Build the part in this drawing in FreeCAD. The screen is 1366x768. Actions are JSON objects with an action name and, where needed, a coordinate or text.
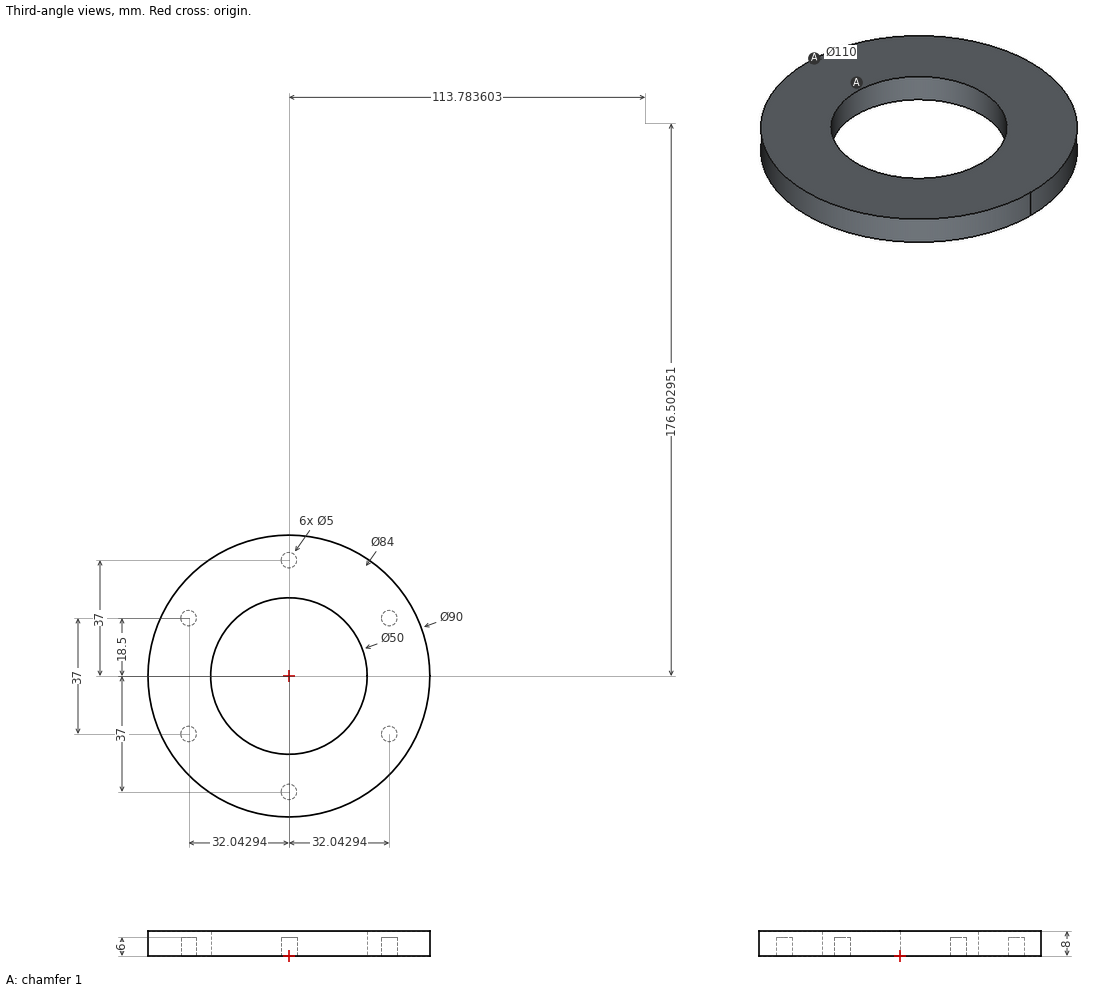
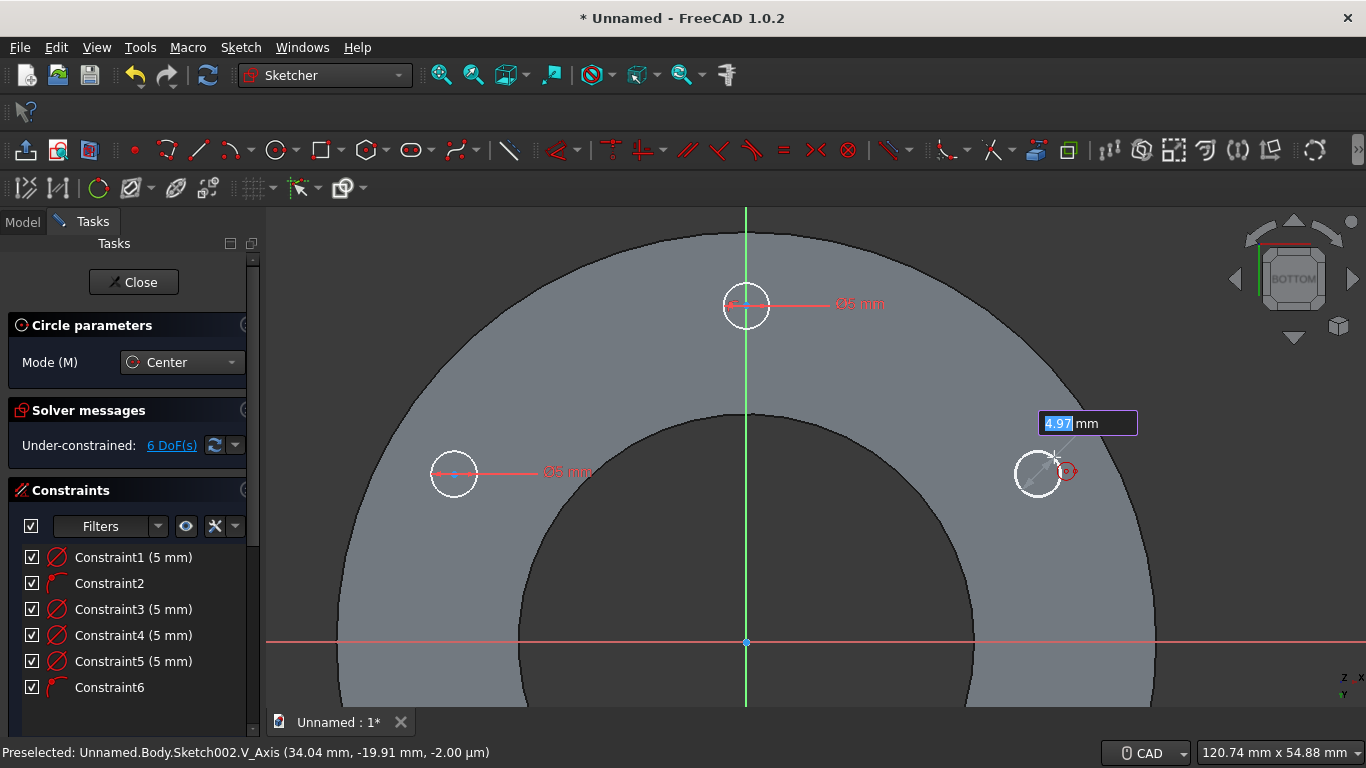
{"action": "type", "text": "5"}
{"action": "key", "text": "Return"}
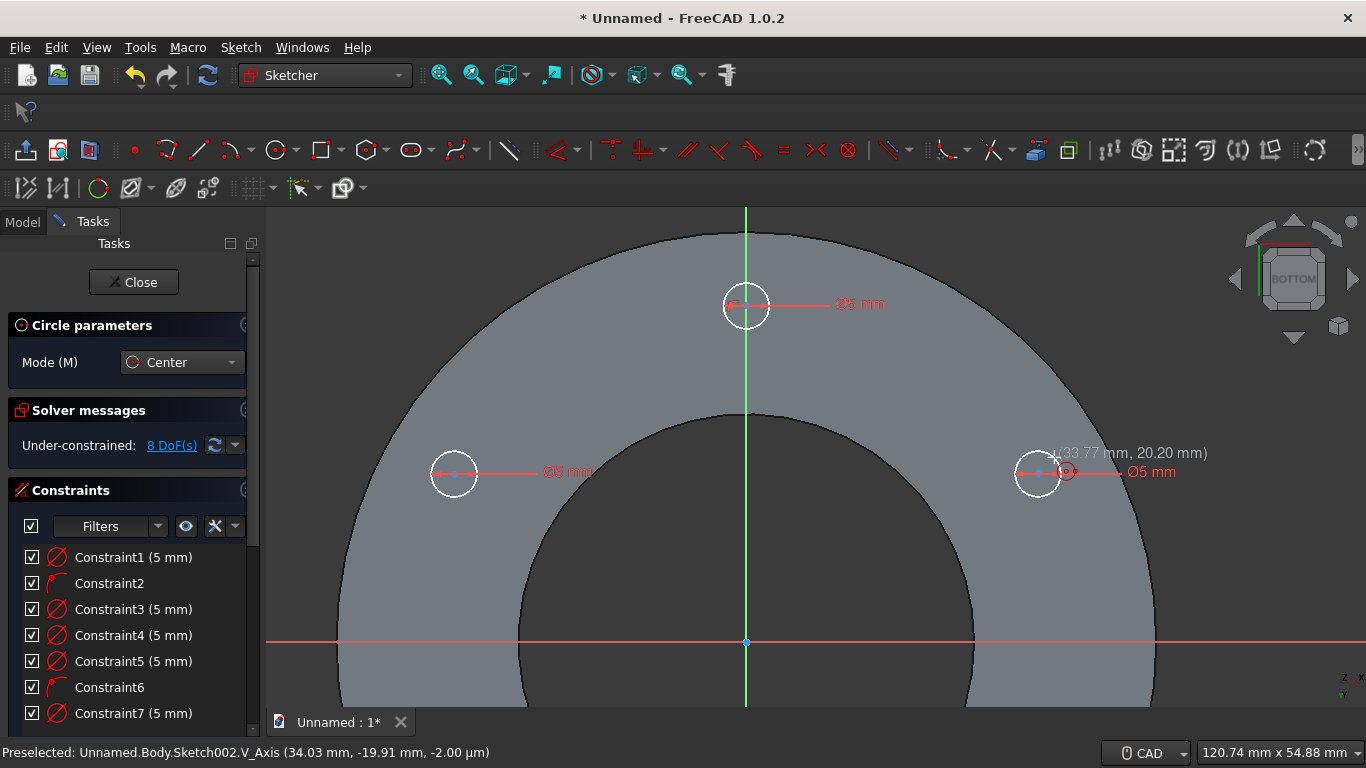
{"action": "scroll", "coordinate": [748, 306], "scroll_direction": "down", "scroll_amount": 4}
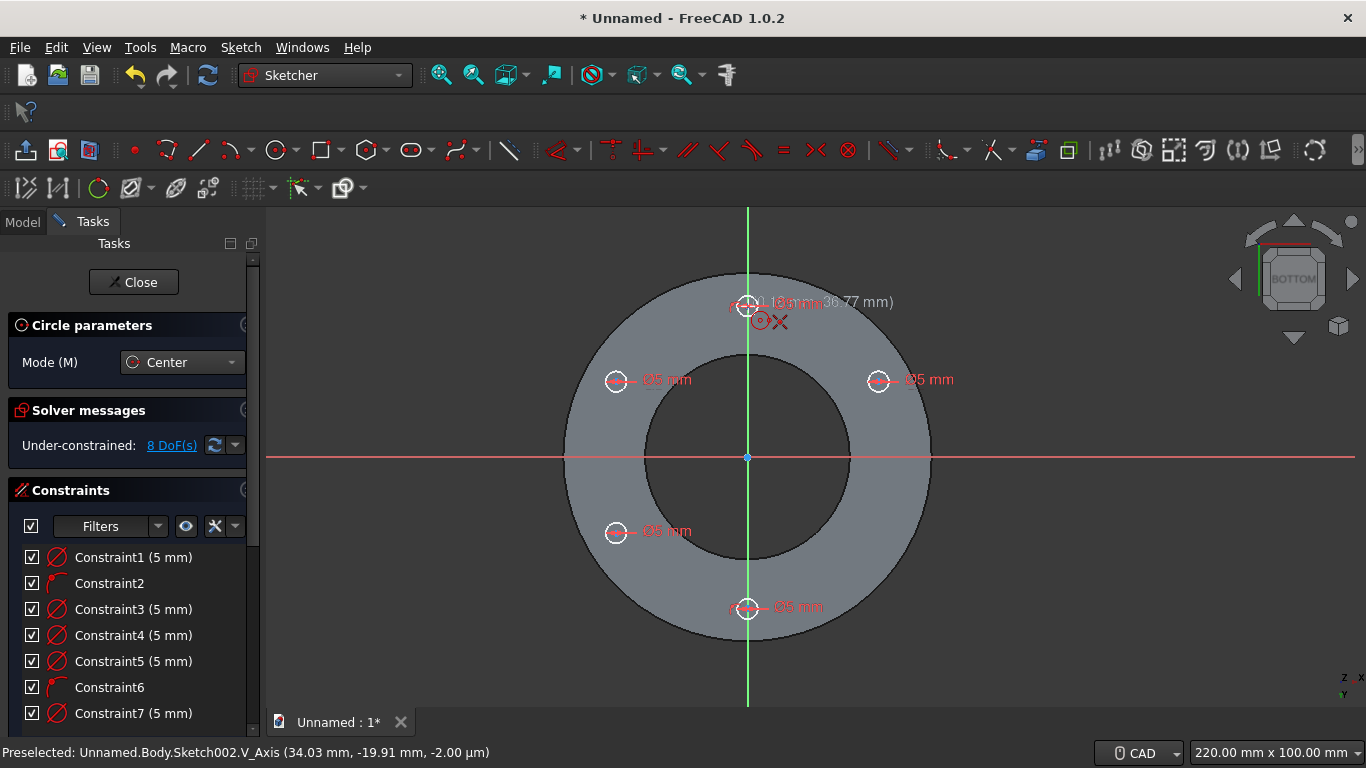
{"action": "scroll", "coordinate": [879, 533], "scroll_direction": "up", "scroll_amount": 4}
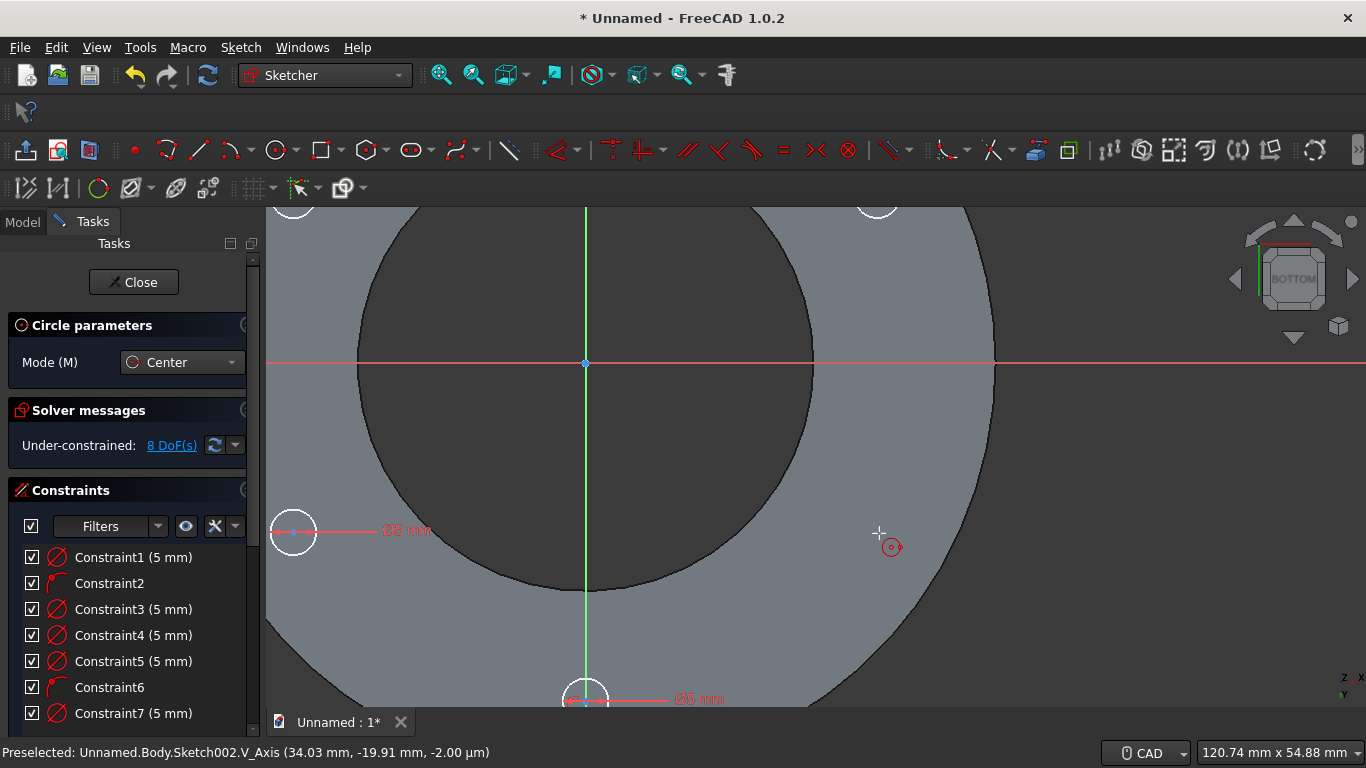
{"action": "left_click", "coordinate": [878, 532]}
{"action": "mouse_move", "coordinate": [894, 516]}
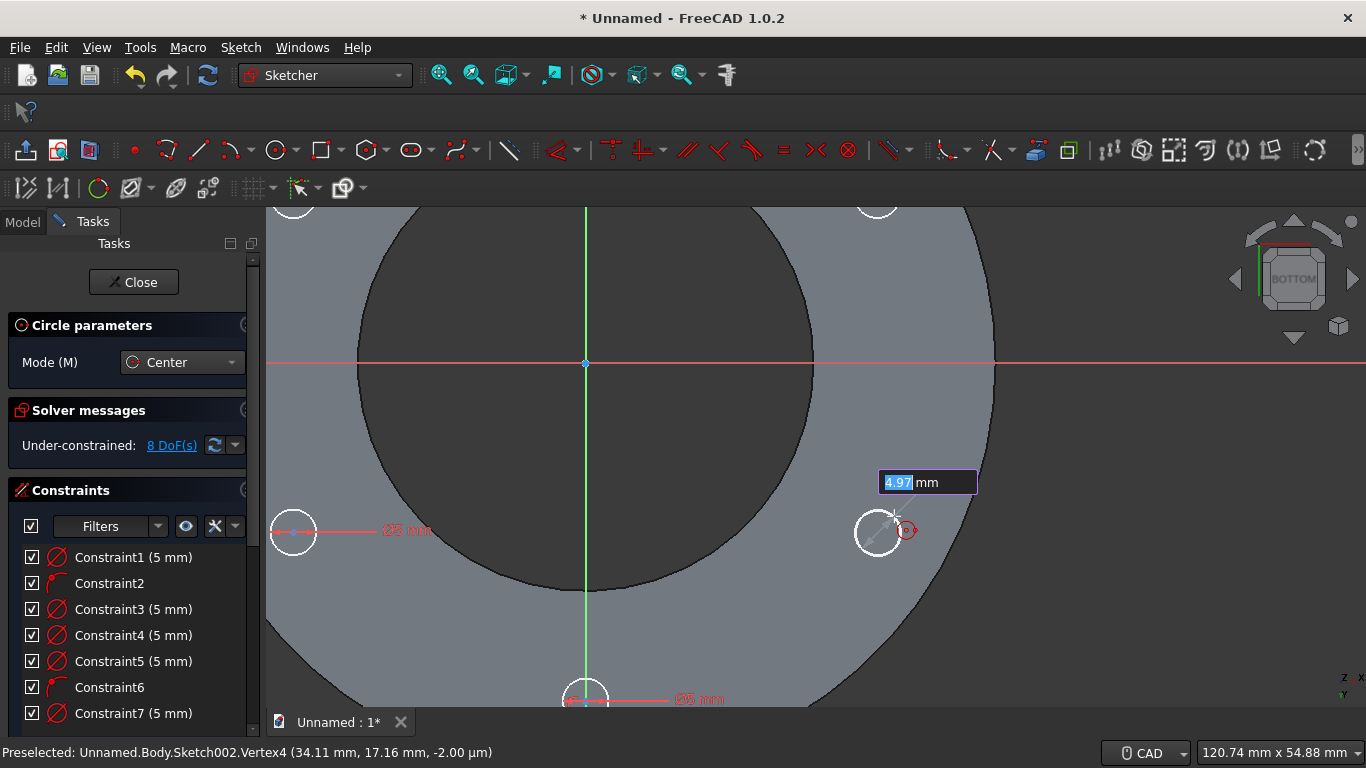
{"action": "type", "text": "5"}
{"action": "key", "text": "Return"}
{"action": "key", "text": "Escape"}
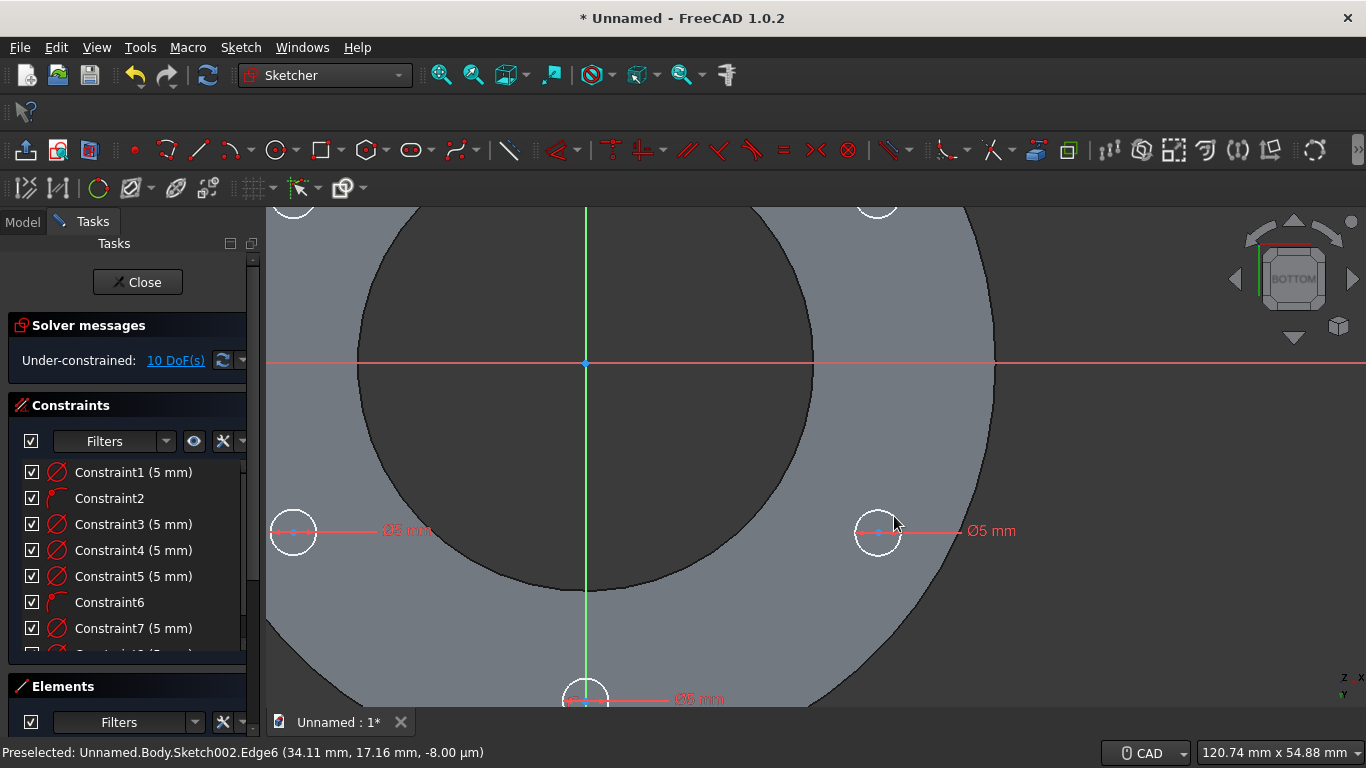
{"action": "key", "text": "d"}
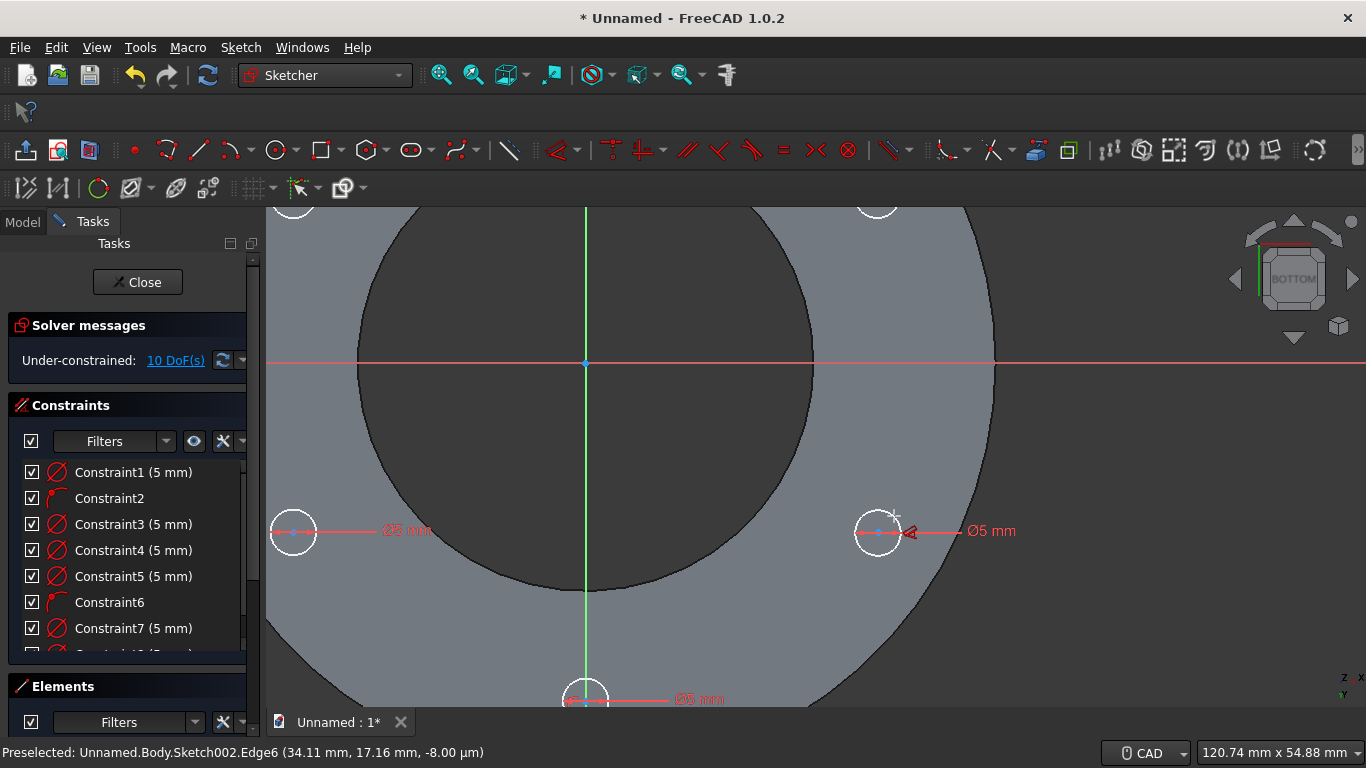
{"action": "scroll", "coordinate": [880, 533], "scroll_direction": "down", "scroll_amount": 4}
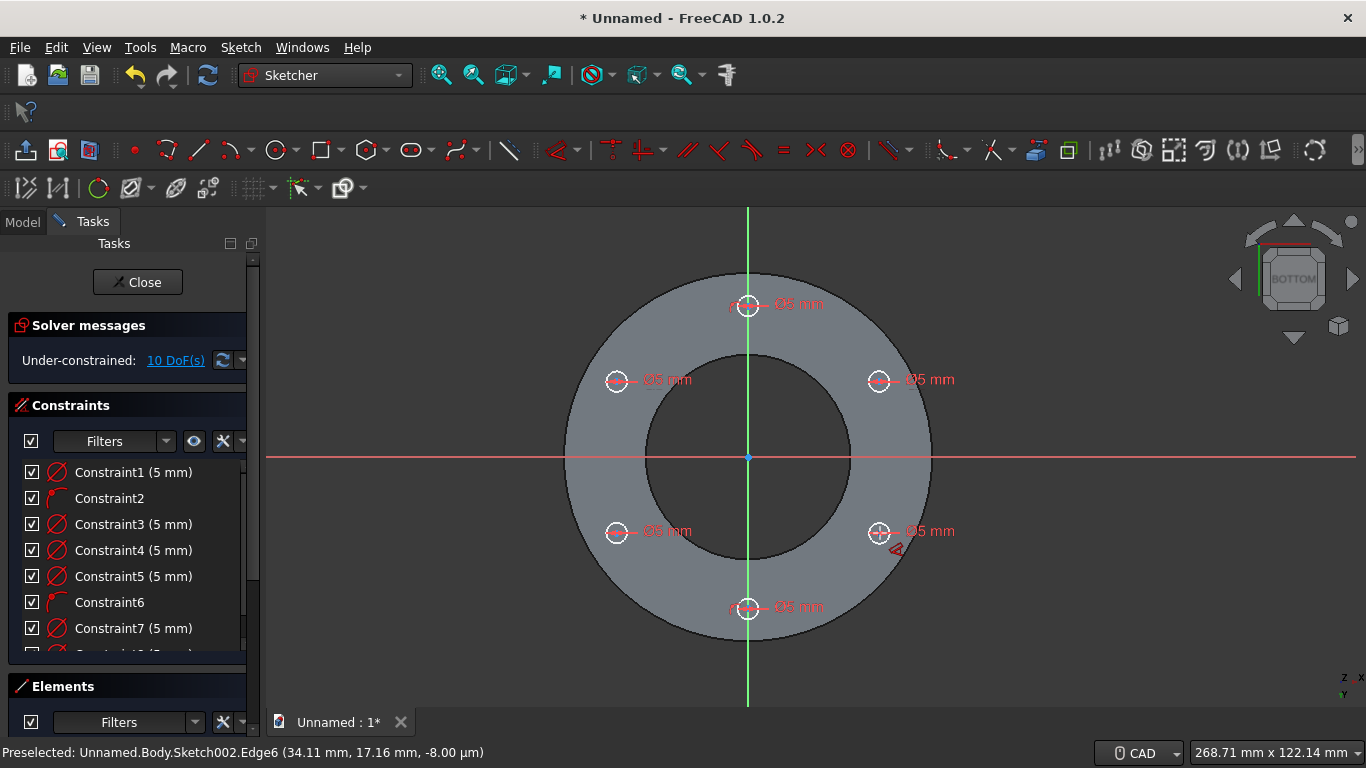
{"action": "left_click", "coordinate": [748, 609]}
{"action": "left_click", "coordinate": [782, 533]}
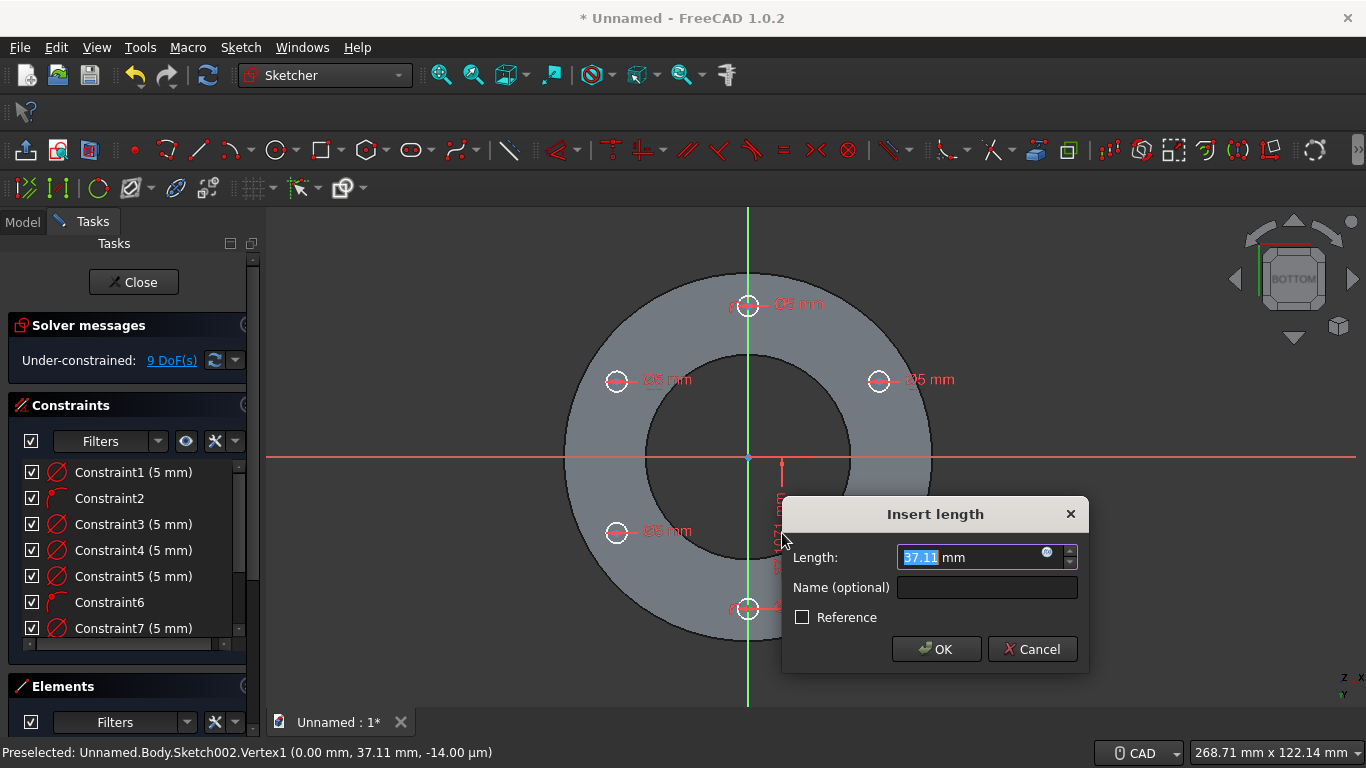
{"action": "type", "text": "37"}
{"action": "key", "text": "Return"}